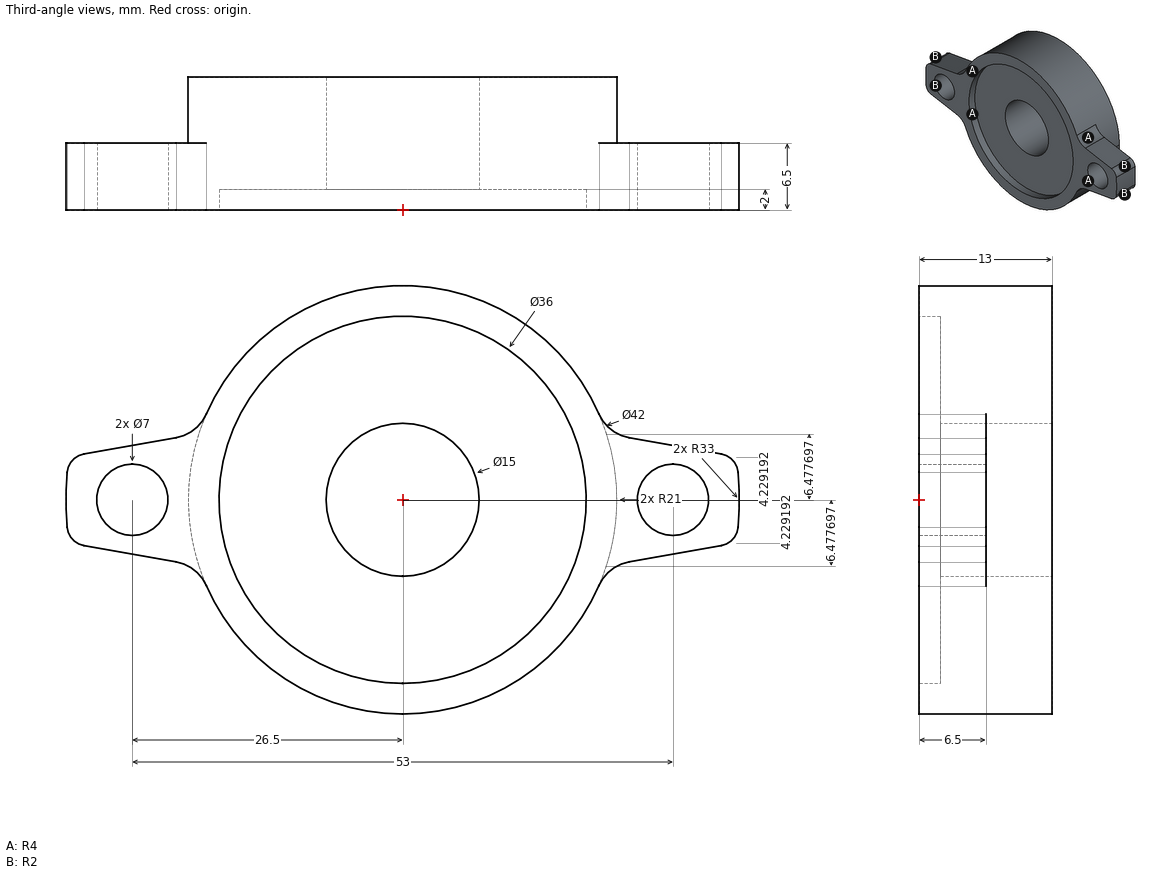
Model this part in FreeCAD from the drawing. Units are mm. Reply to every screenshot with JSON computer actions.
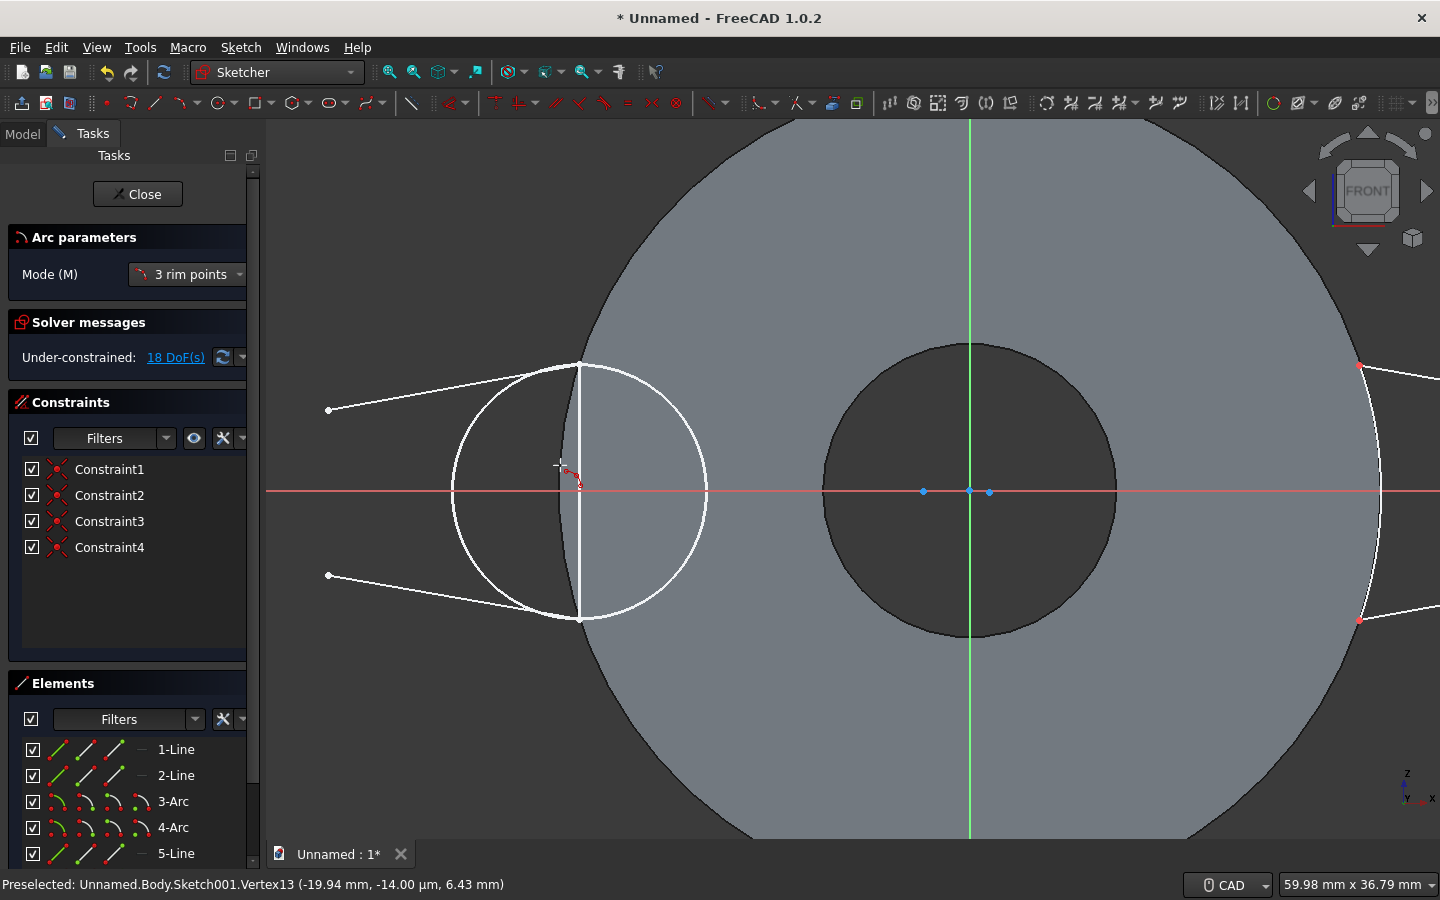
{"action": "left_click", "coordinate": [560, 465]}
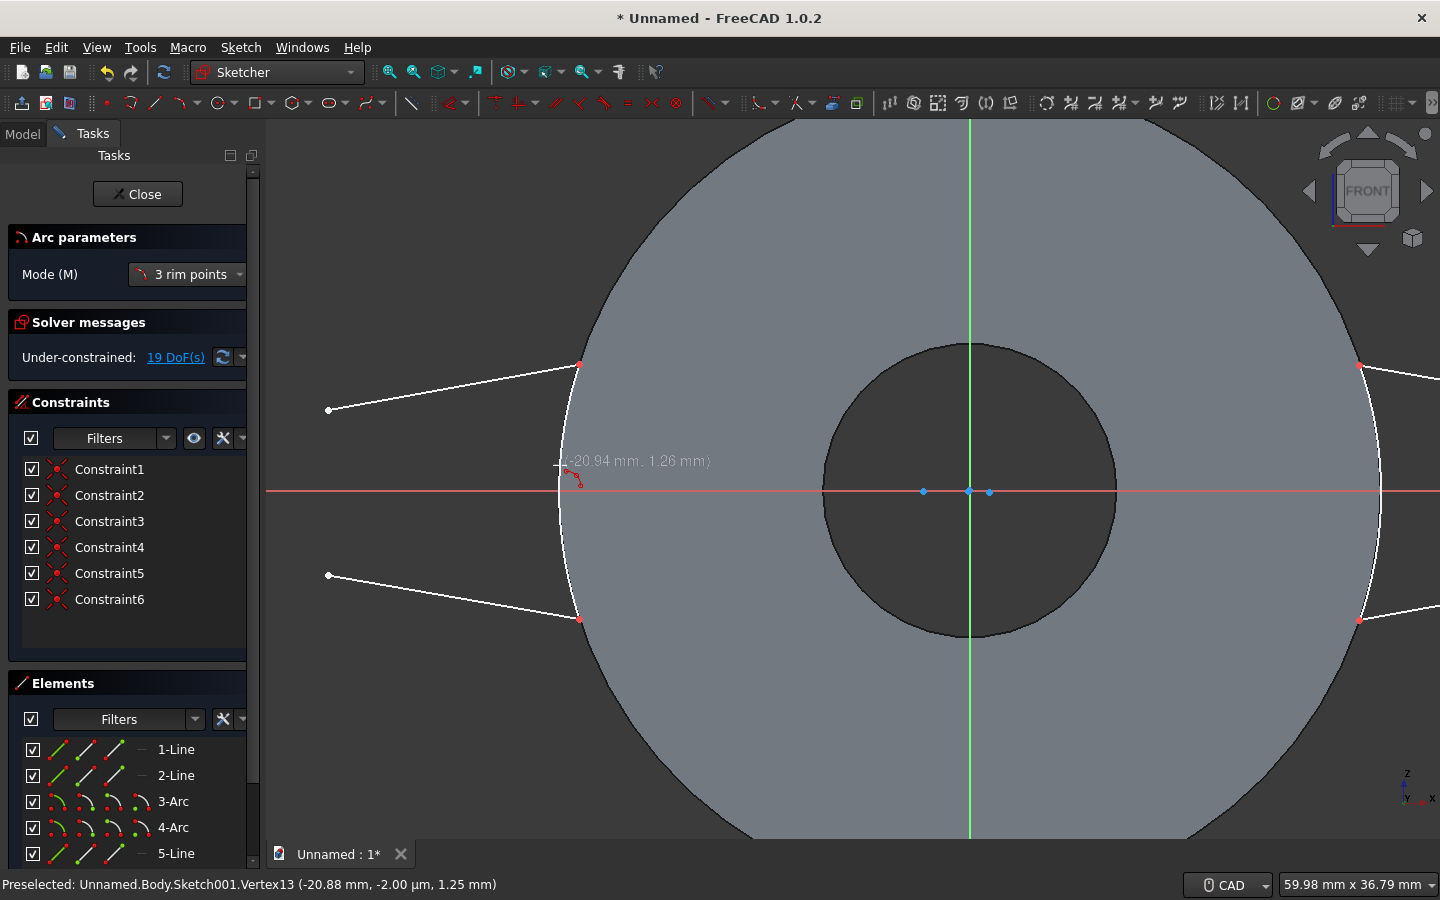
{"action": "left_click", "coordinate": [329, 410]}
{"action": "left_click", "coordinate": [329, 576]}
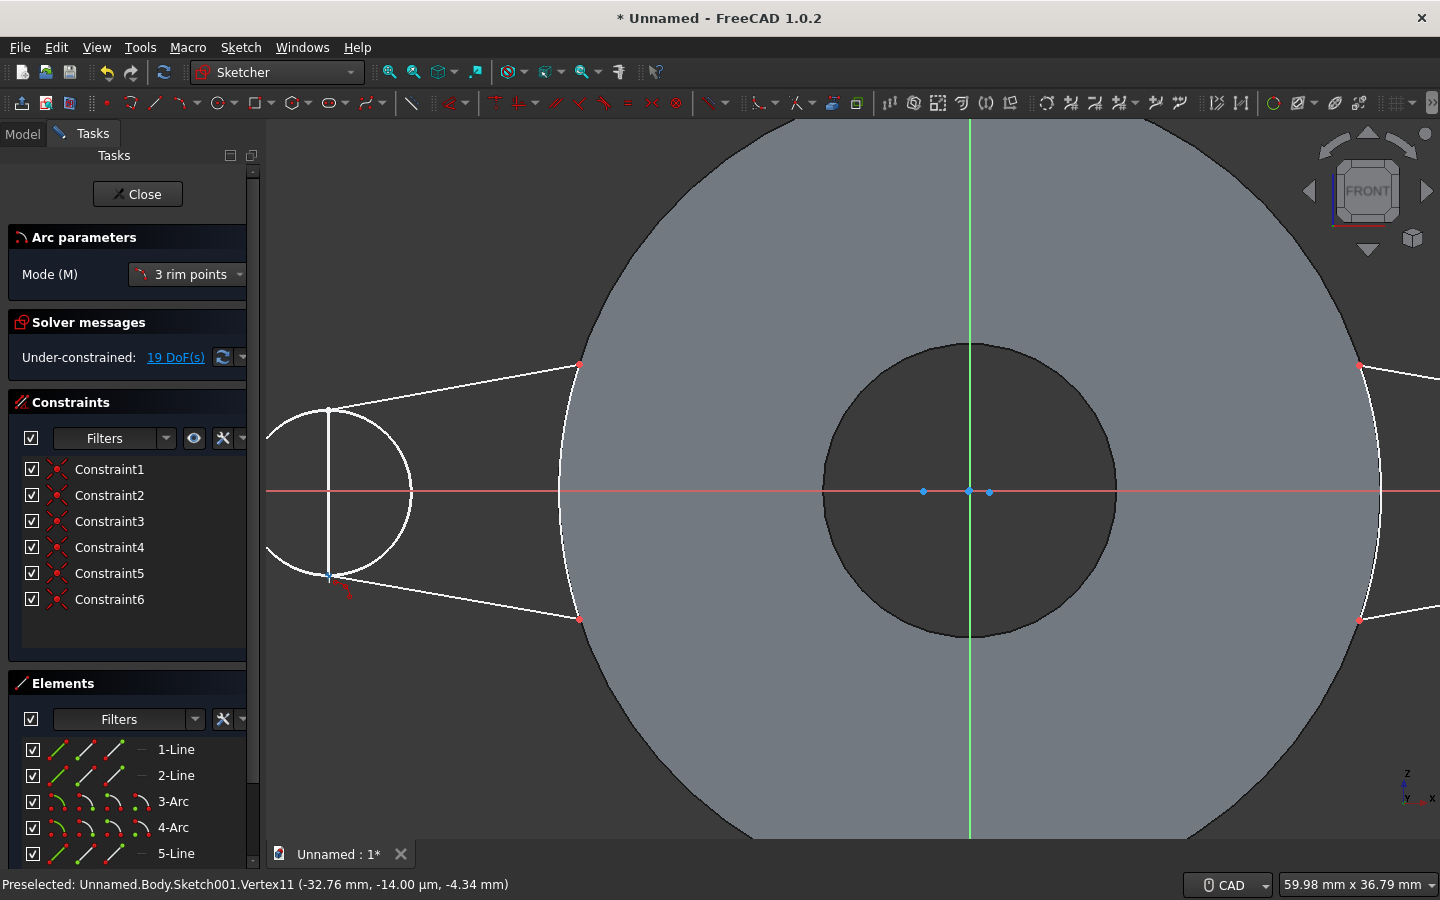
{"action": "scroll", "coordinate": [324, 474], "scroll_direction": "up", "scroll_amount": 6}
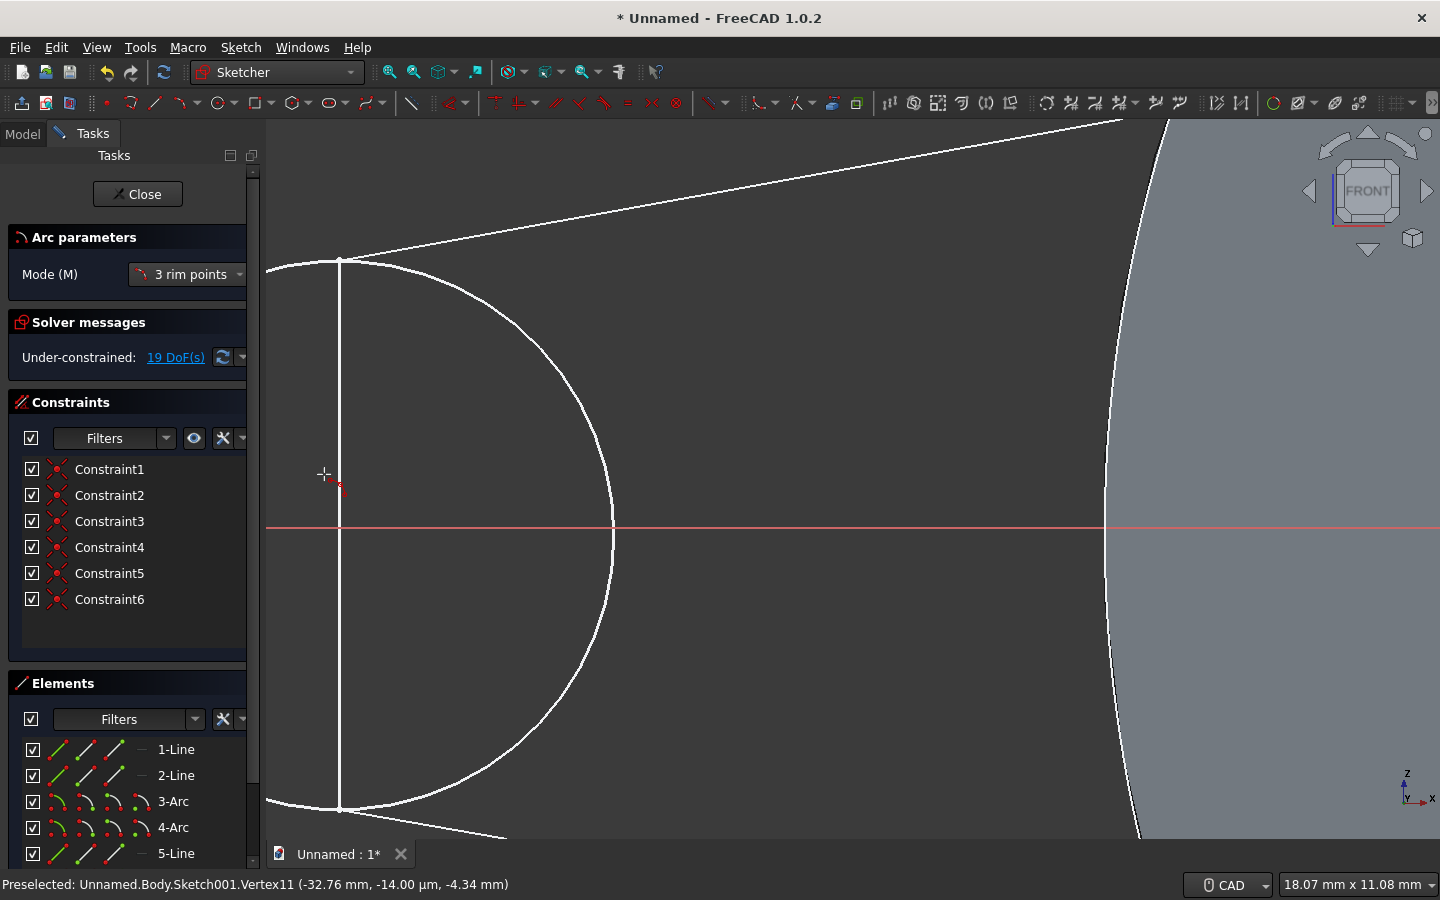
{"action": "left_click", "coordinate": [324, 473]}
{"action": "key", "text": "Escape"}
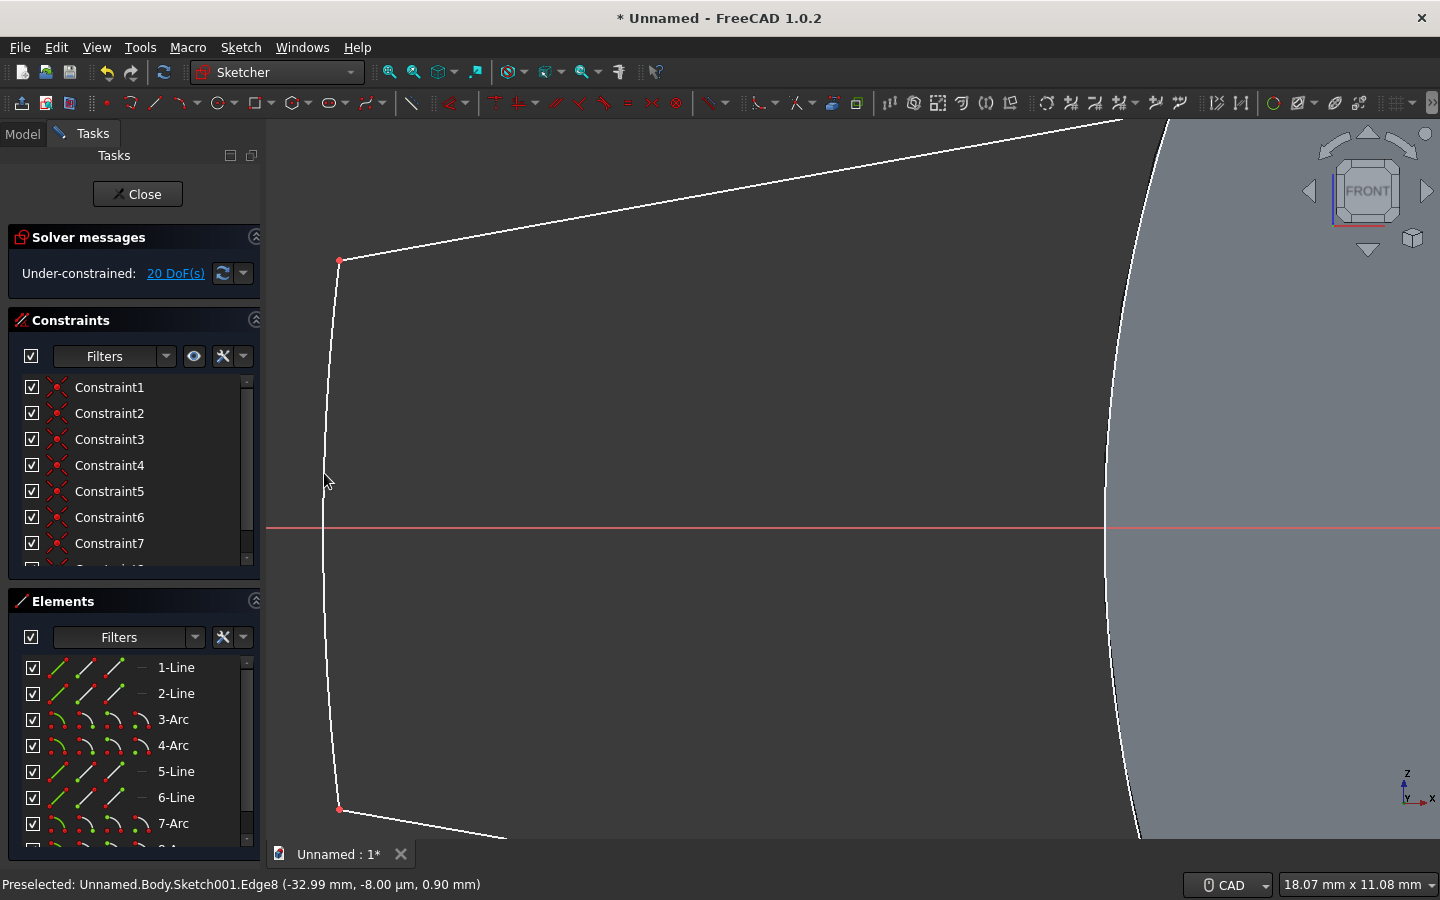
{"action": "scroll", "coordinate": [451, 469], "scroll_direction": "down", "scroll_amount": 9}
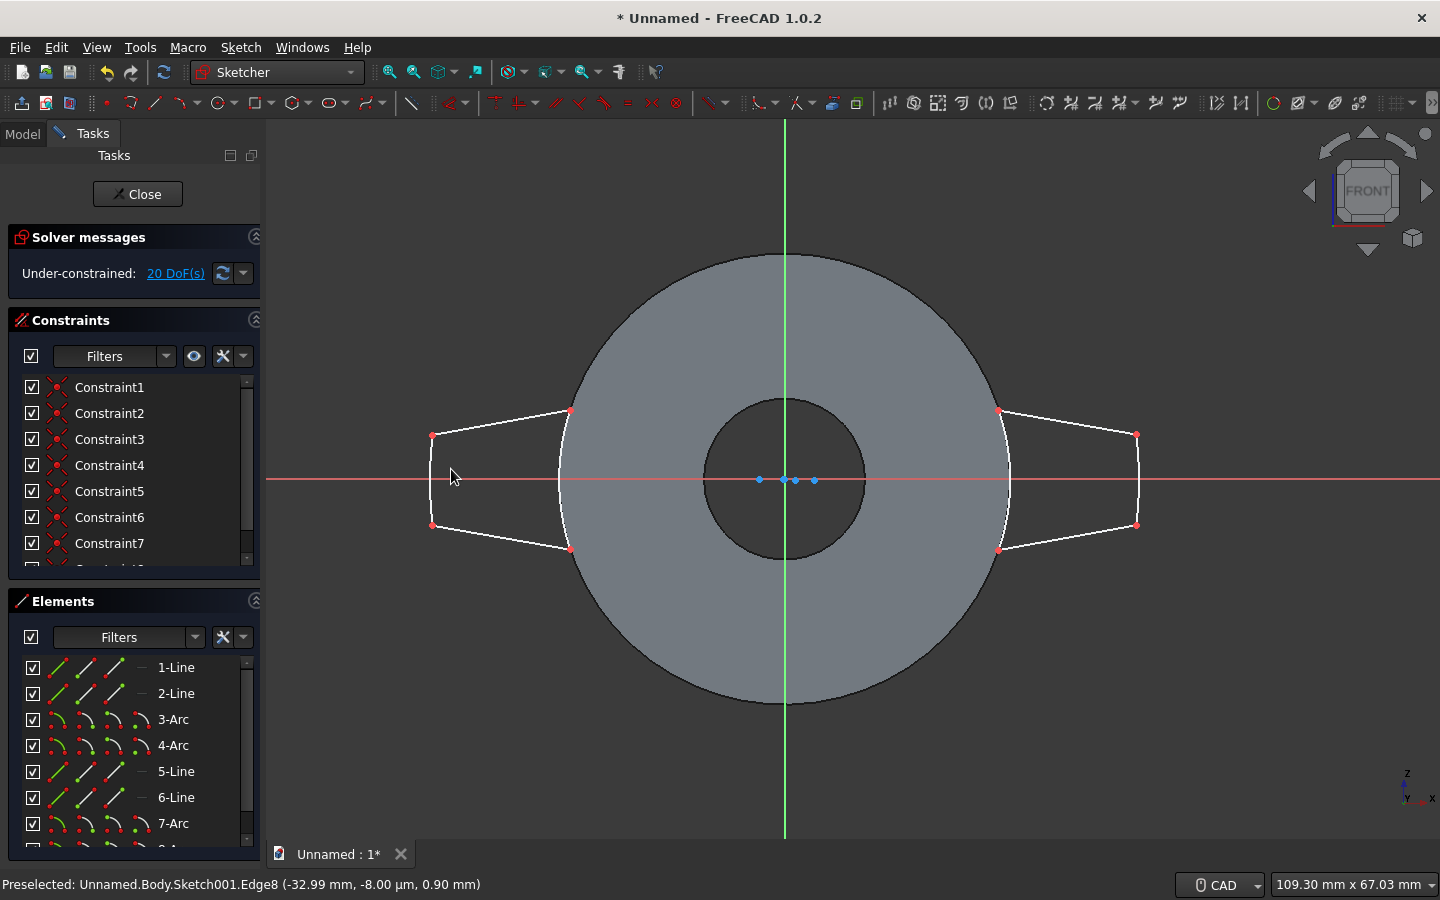
{"action": "left_click", "coordinate": [1008, 509]}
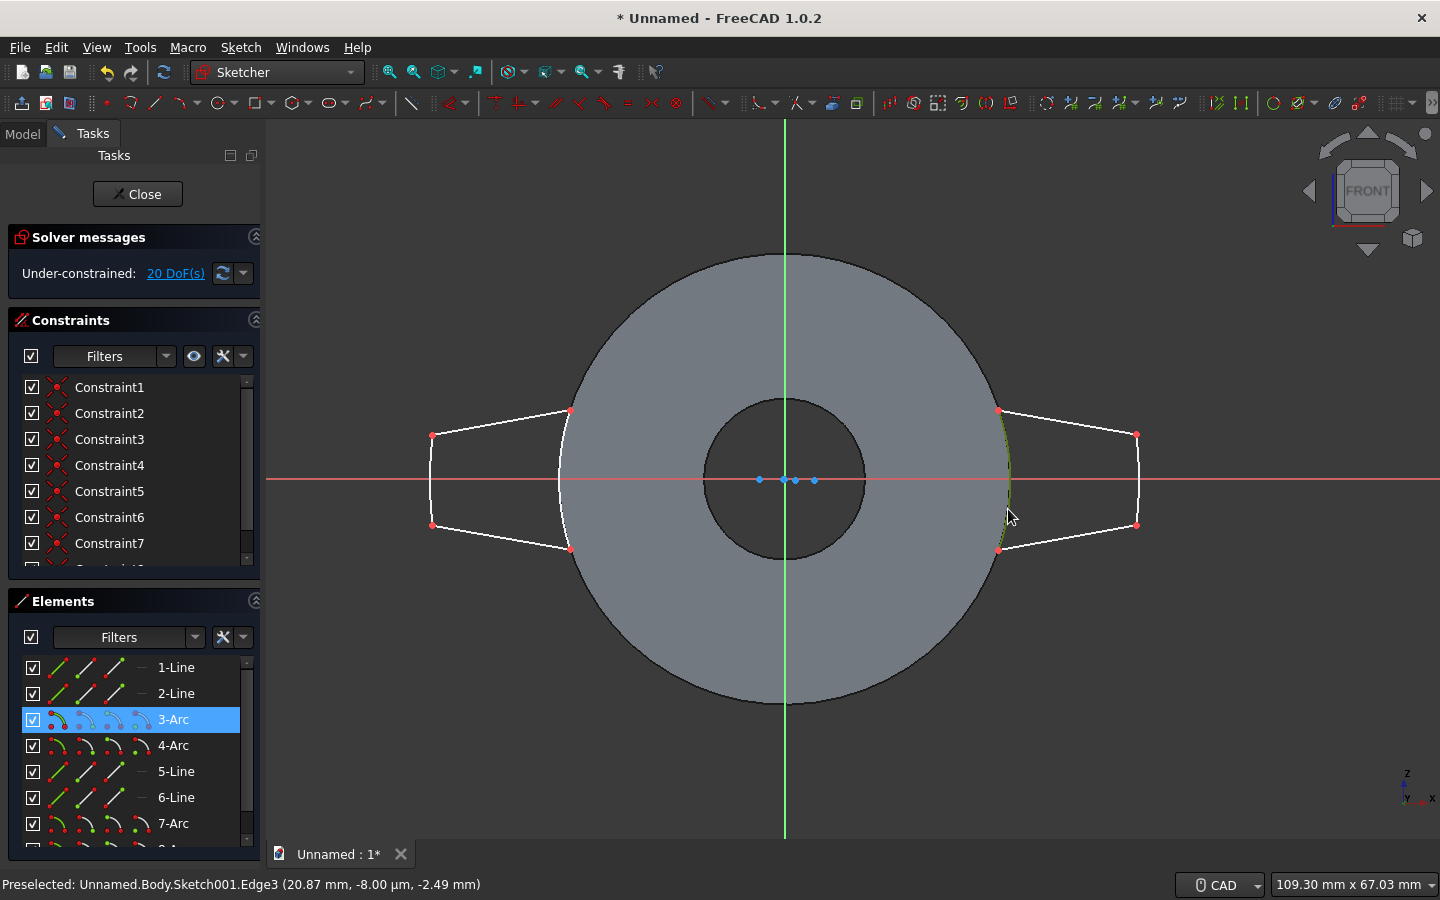
{"action": "left_click", "coordinate": [1138, 498]}